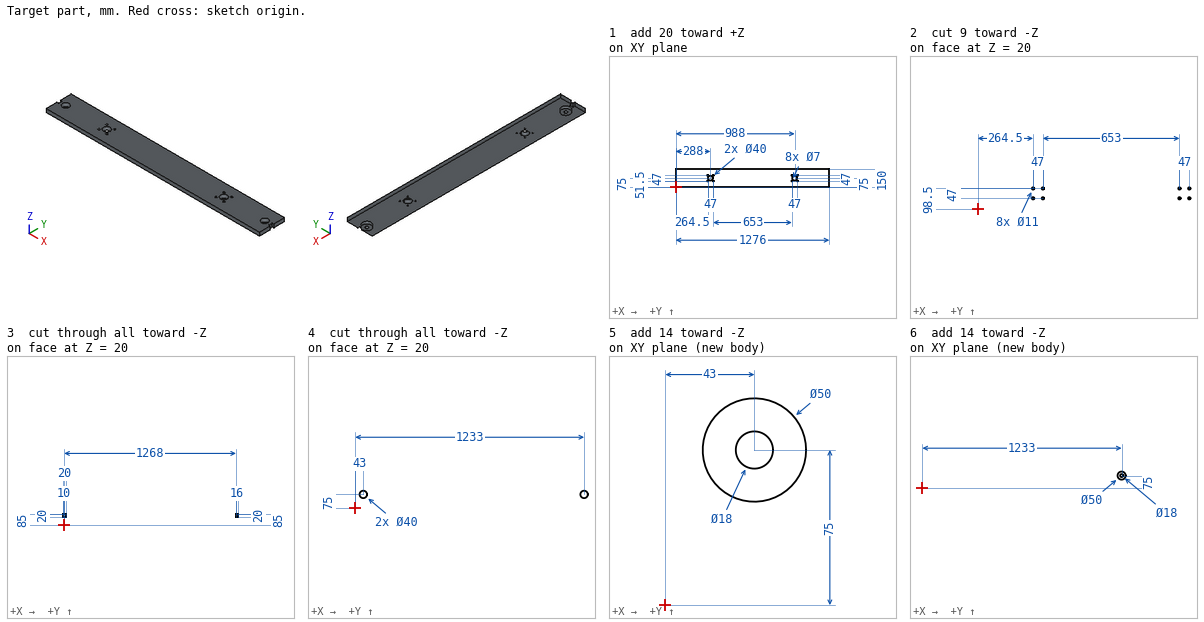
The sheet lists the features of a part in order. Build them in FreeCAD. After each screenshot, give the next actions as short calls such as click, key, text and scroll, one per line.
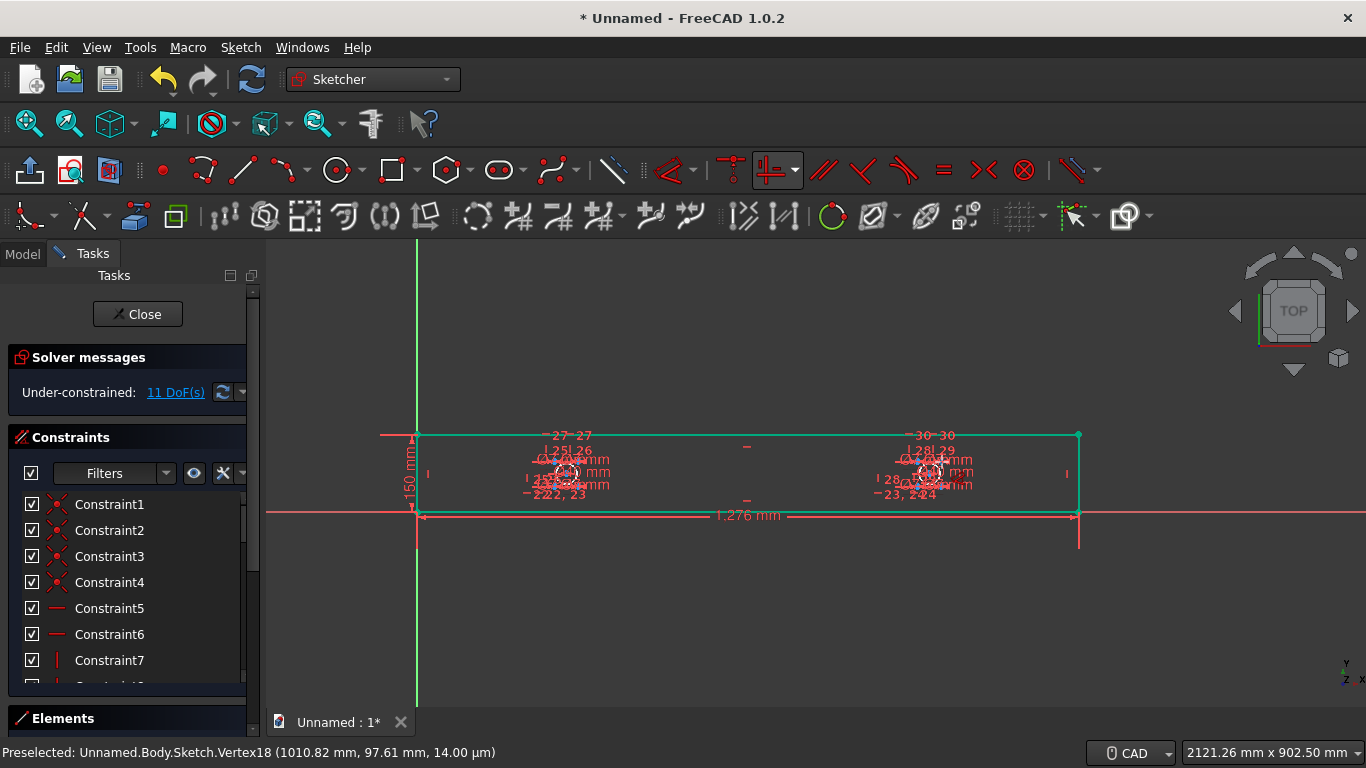
click(566, 474)
click(383, 493)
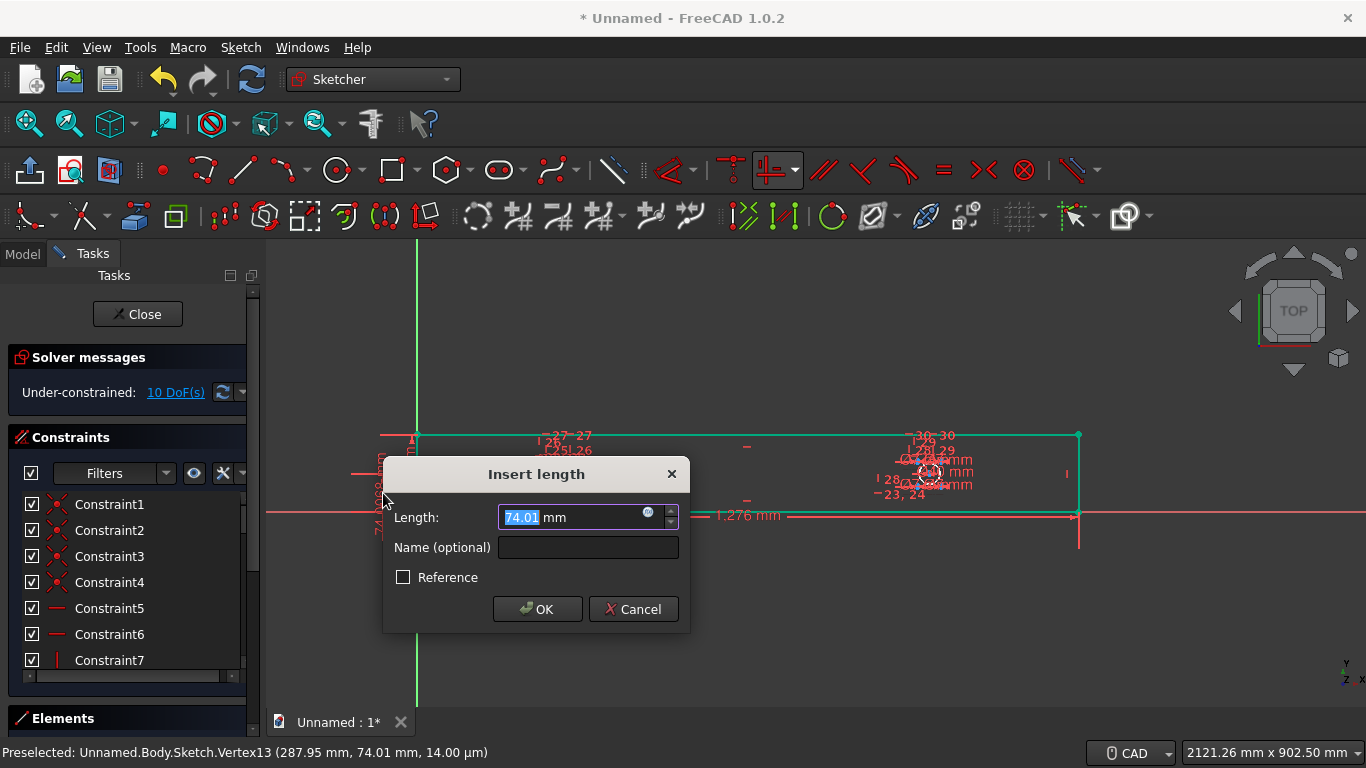
text(75)
key(Return)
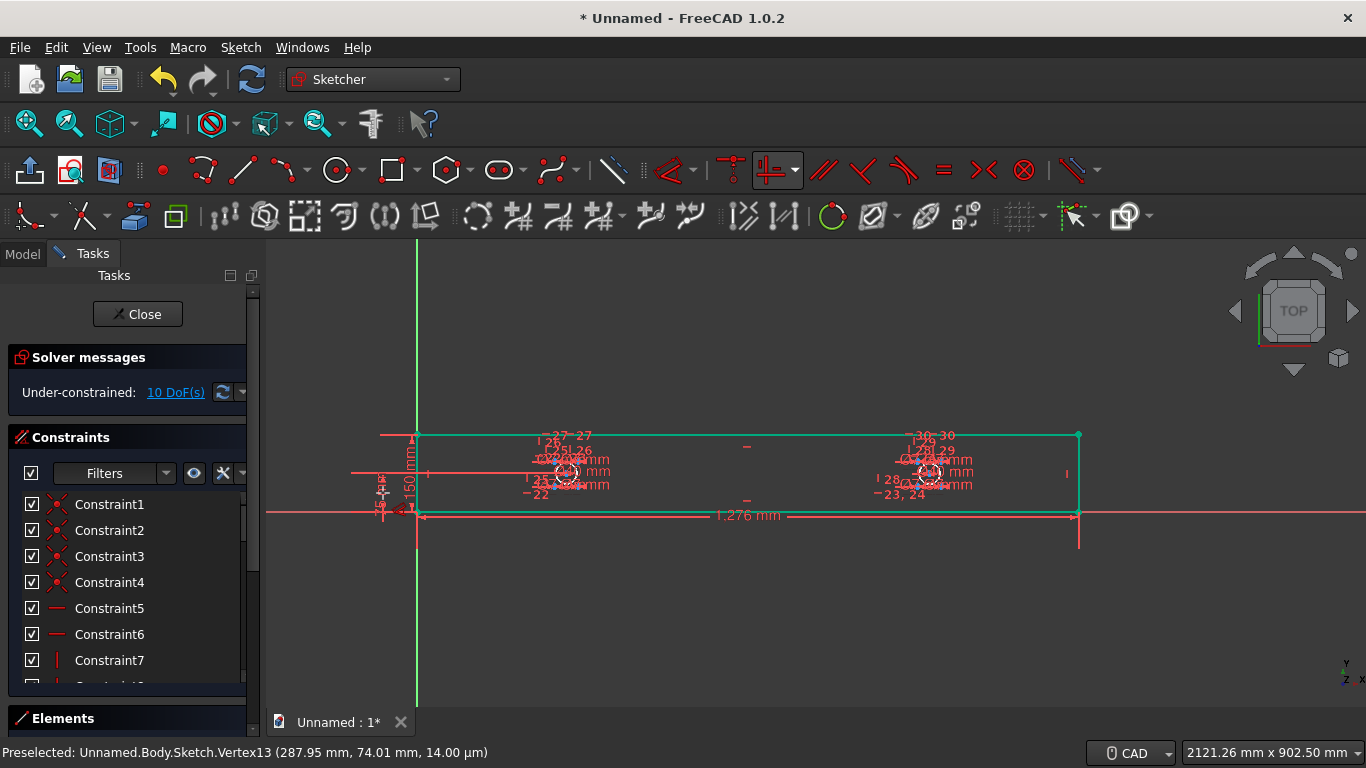
click(930, 474)
click(964, 493)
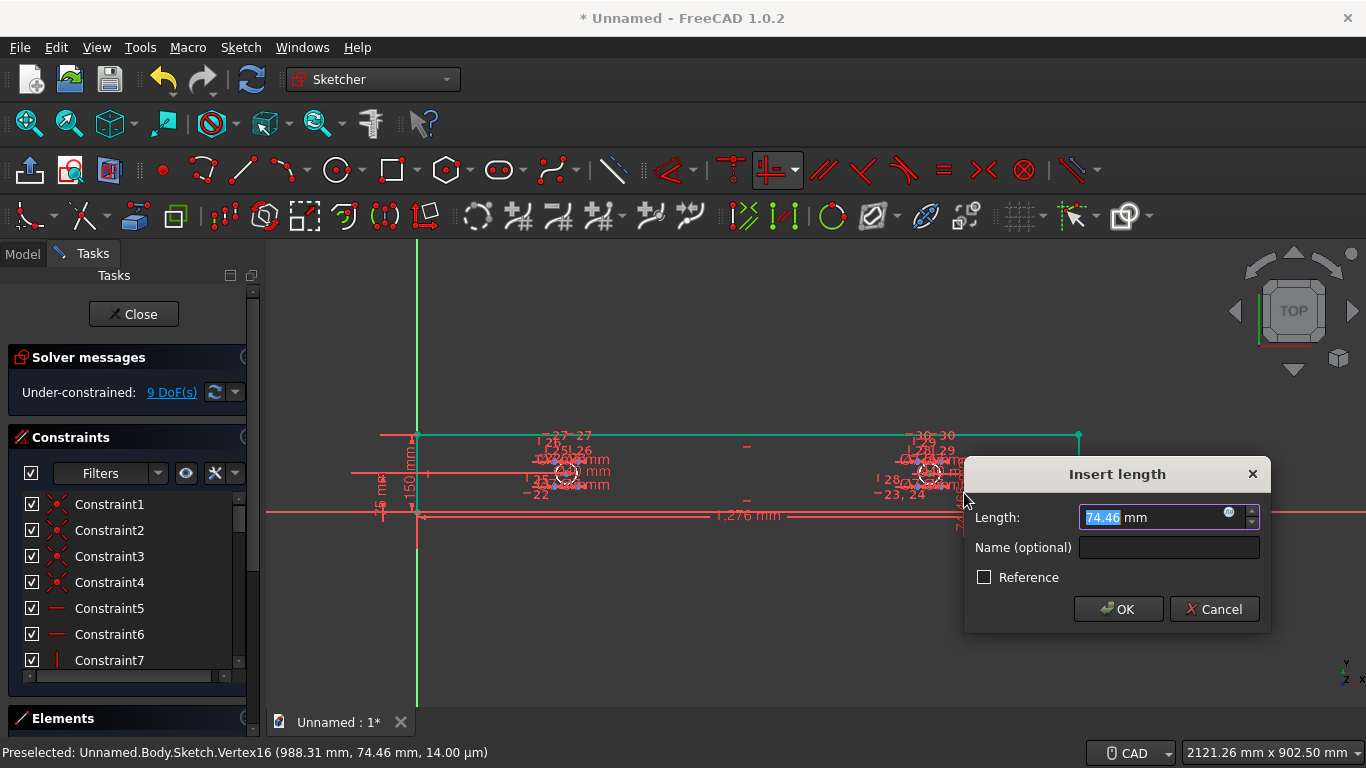
text(75)
key(Return)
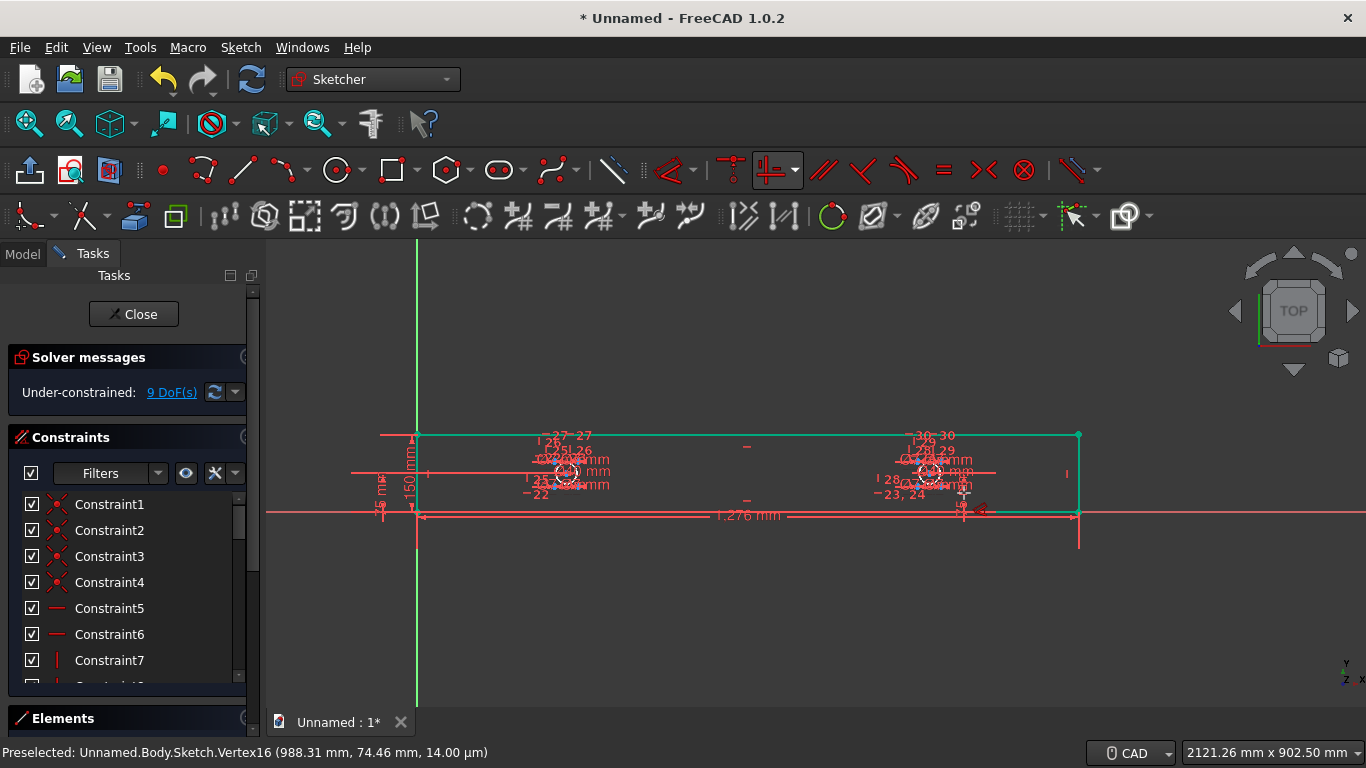
click(566, 473)
click(492, 546)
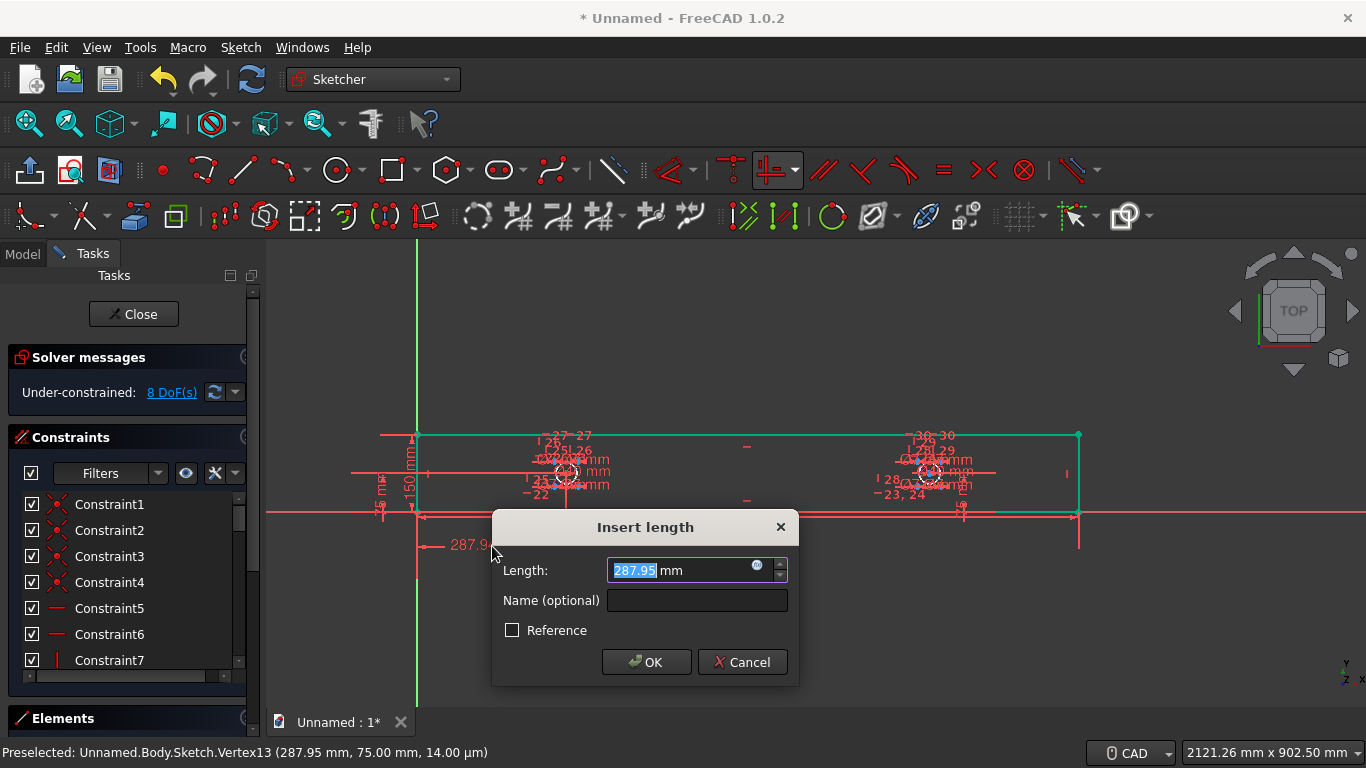
text(288)
key(Return)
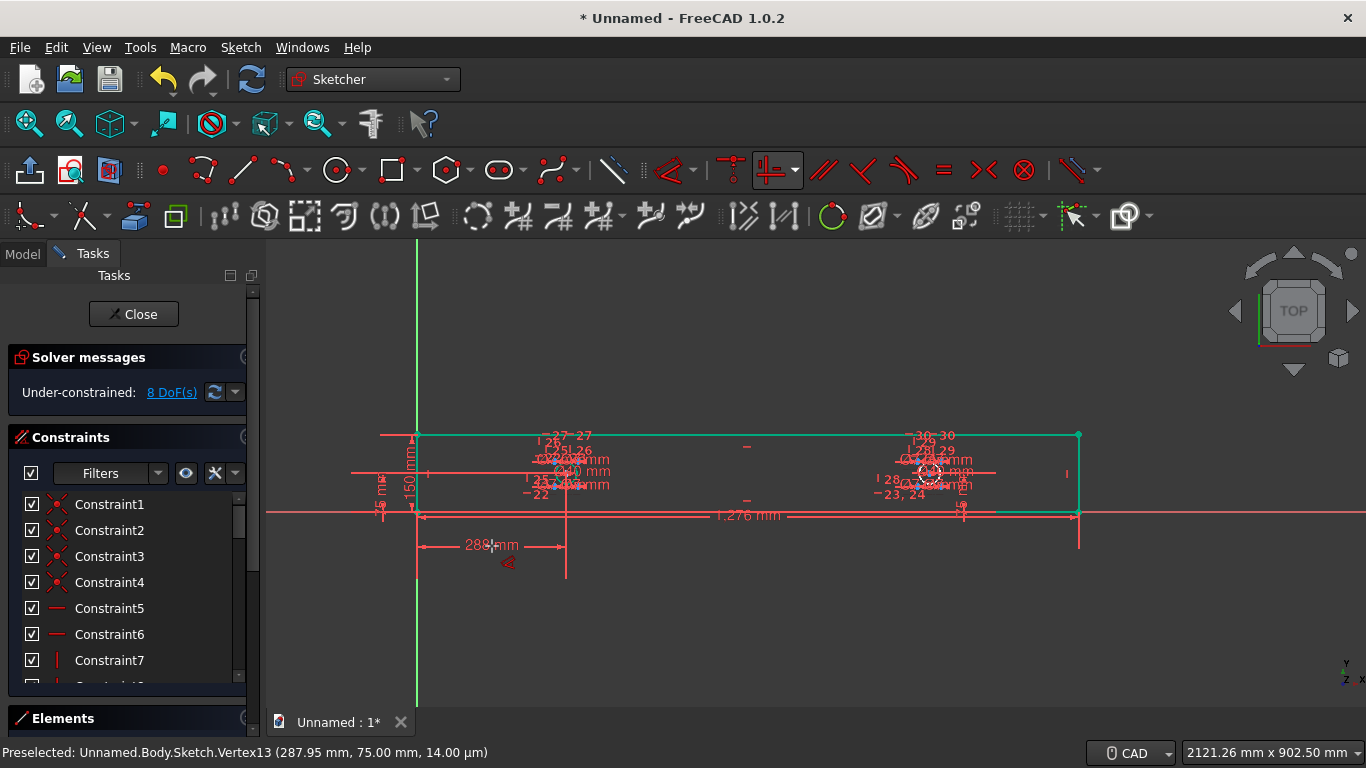
click(930, 473)
click(673, 546)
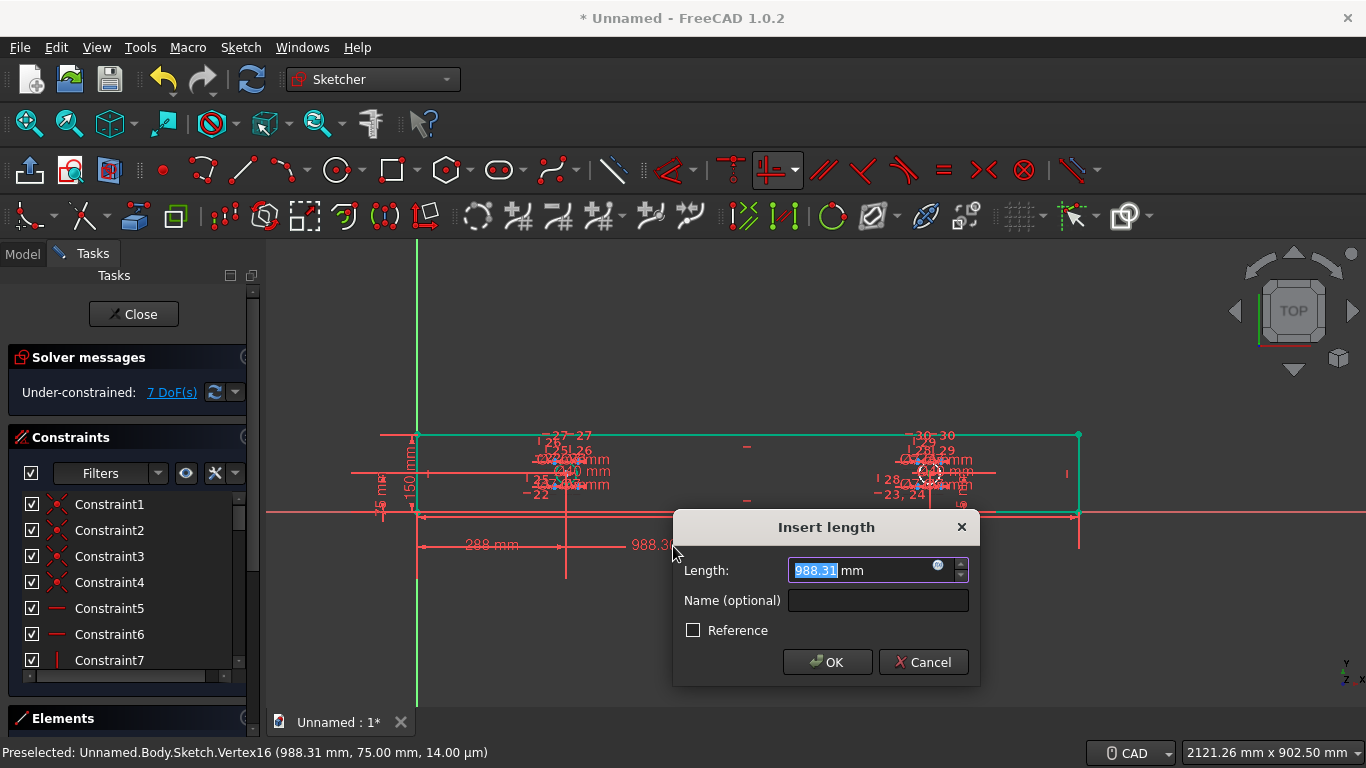
text(988)
key(Return)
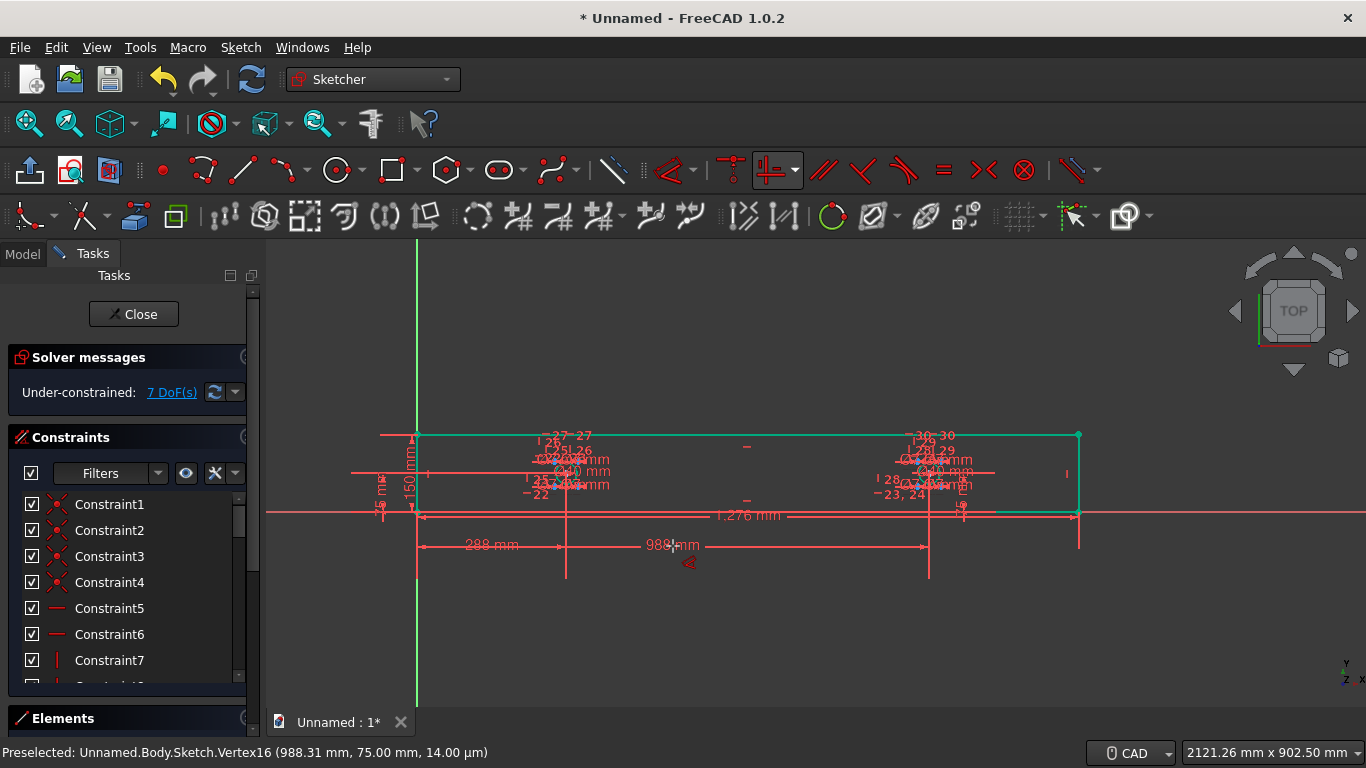
scroll(554, 487, up, 3)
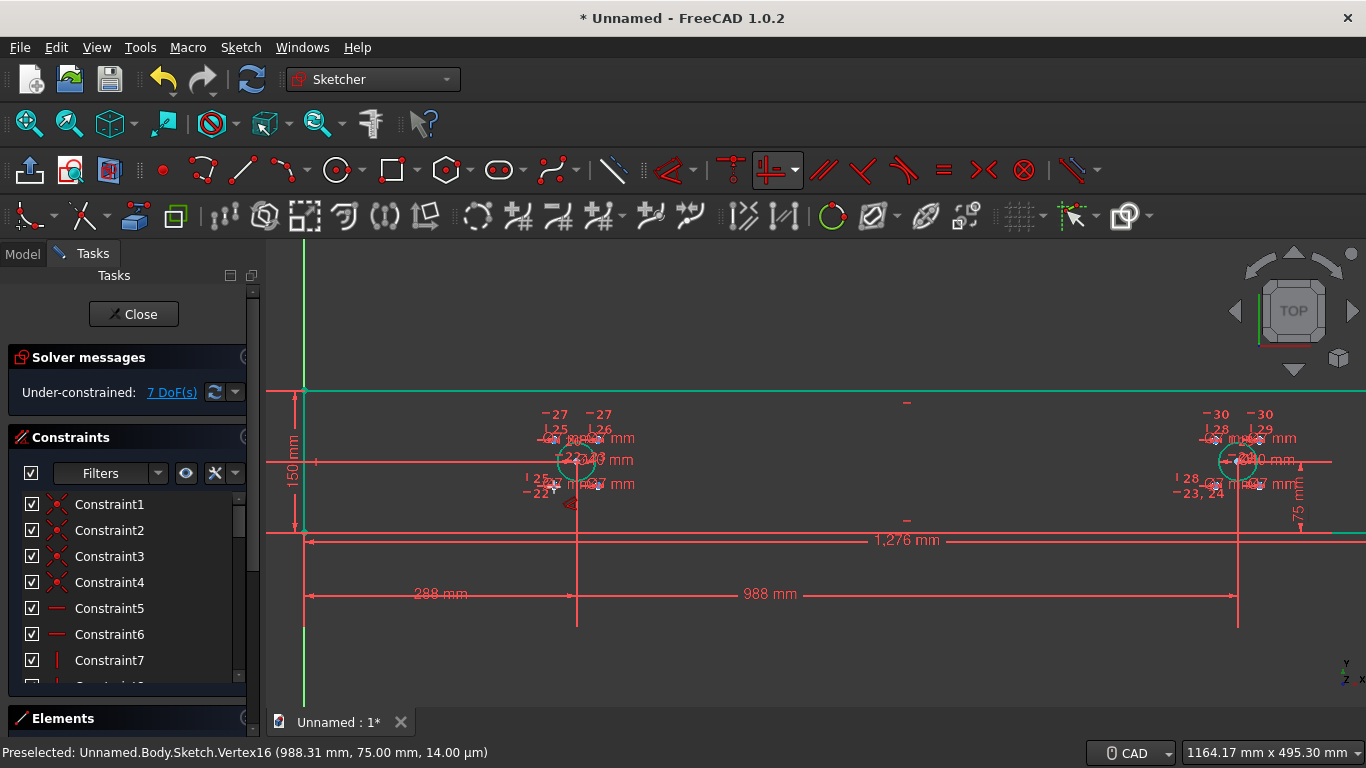
click(554, 486)